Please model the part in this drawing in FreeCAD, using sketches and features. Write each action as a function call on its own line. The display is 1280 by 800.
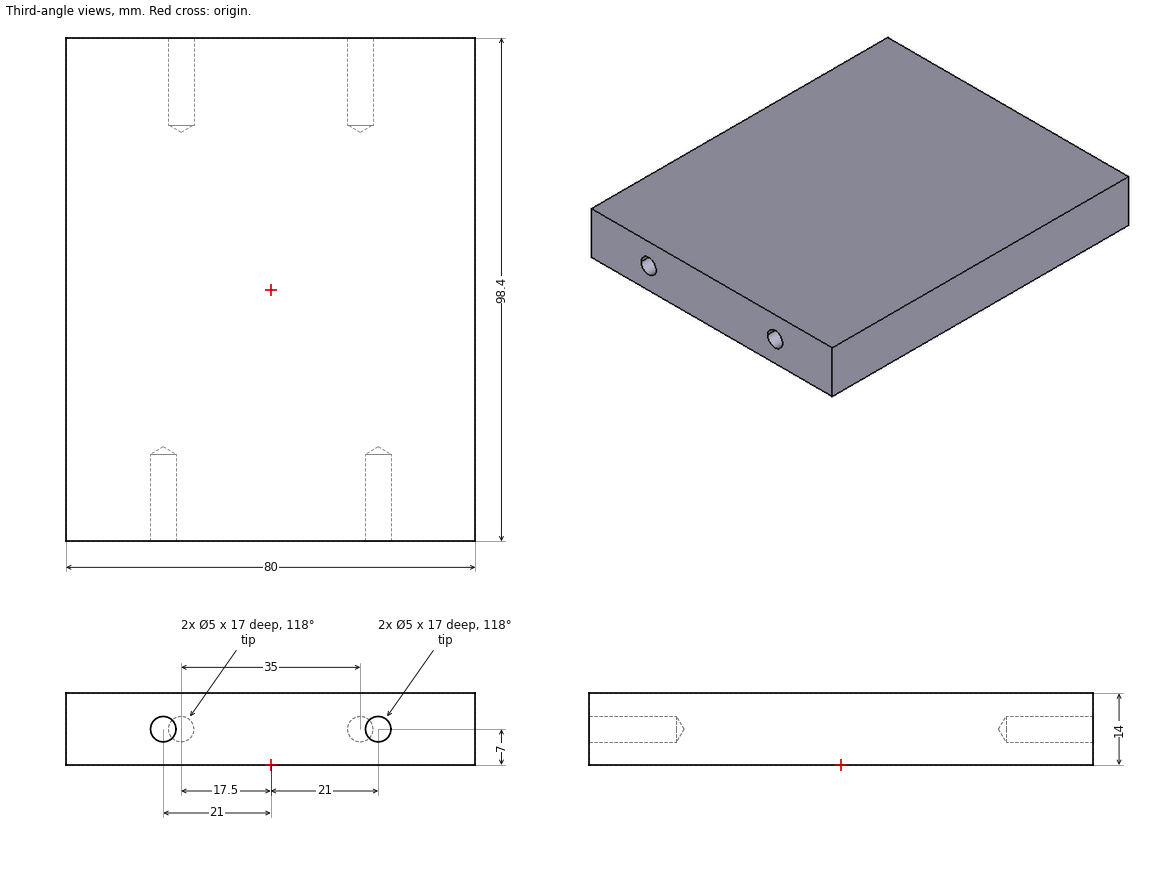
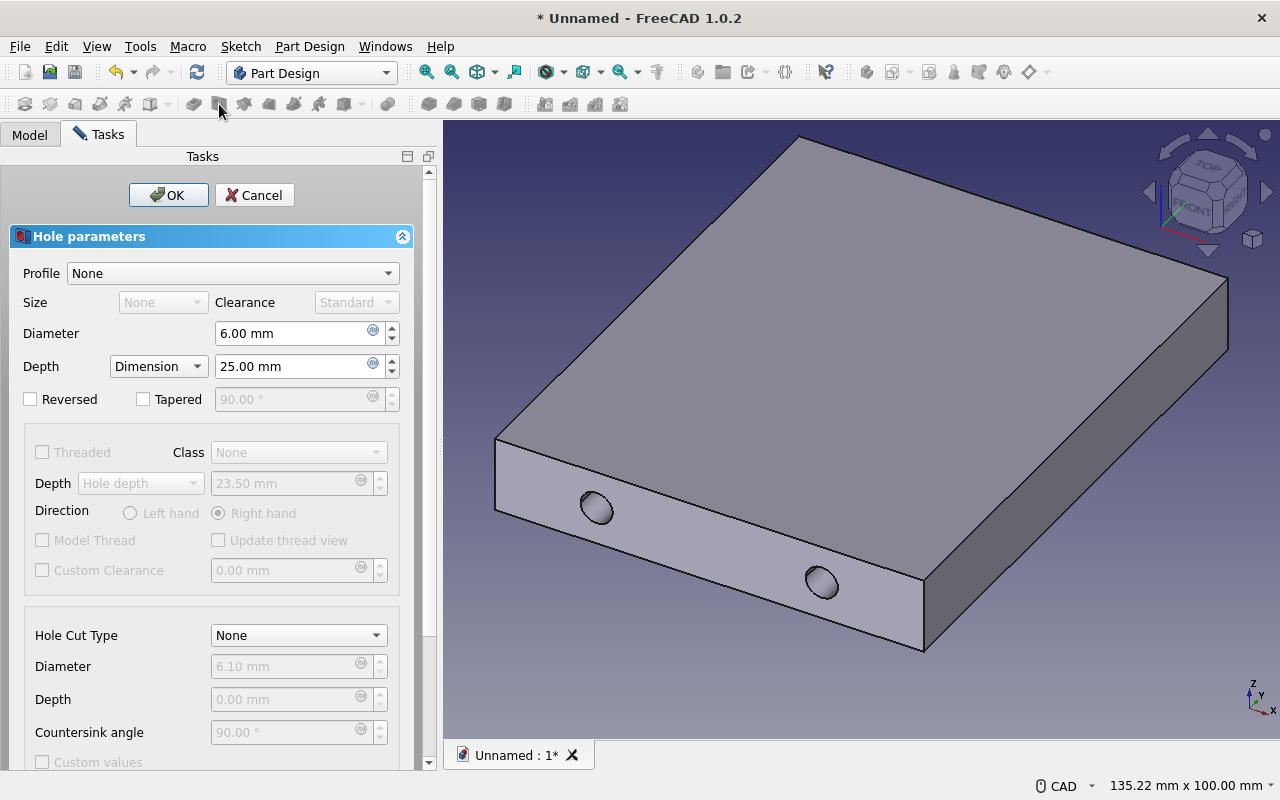
triple_click(300, 334)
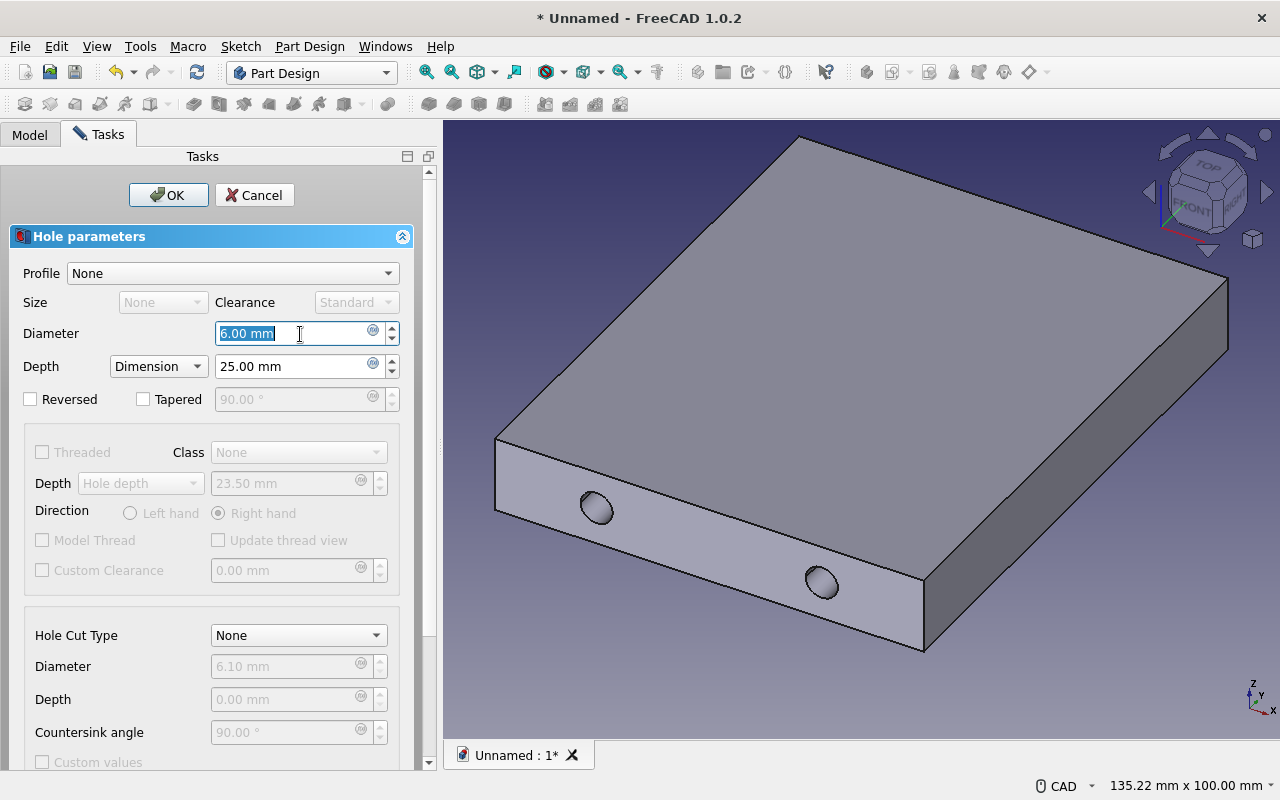
text(5)
key(Tab)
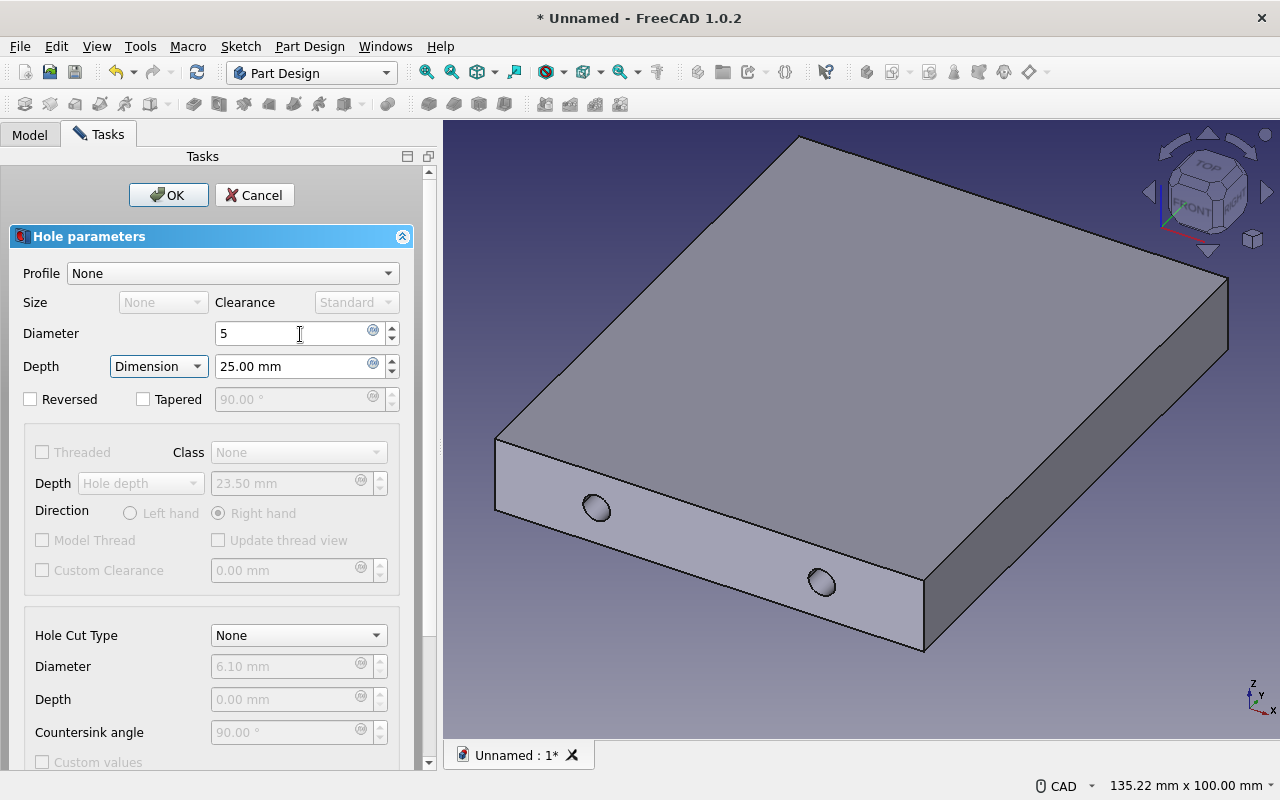
triple_click(300, 366)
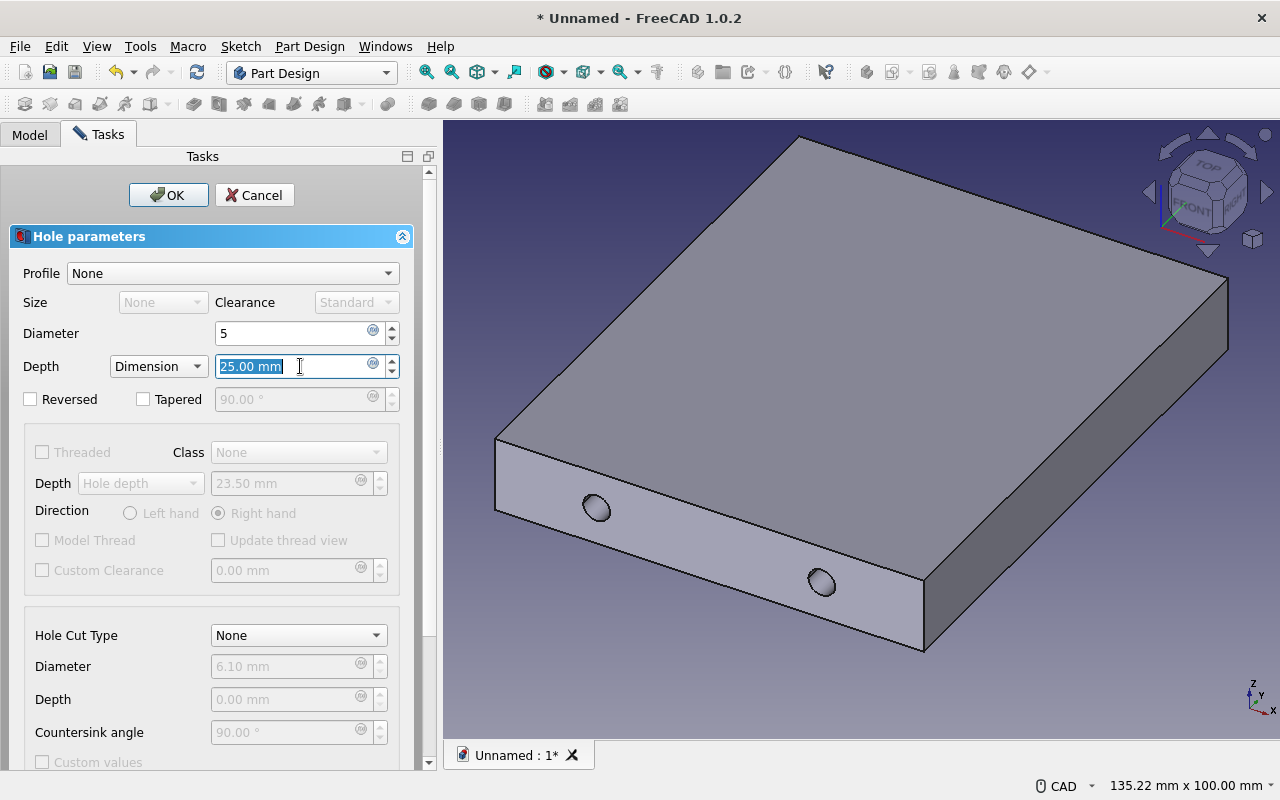
text(17)
key(Tab)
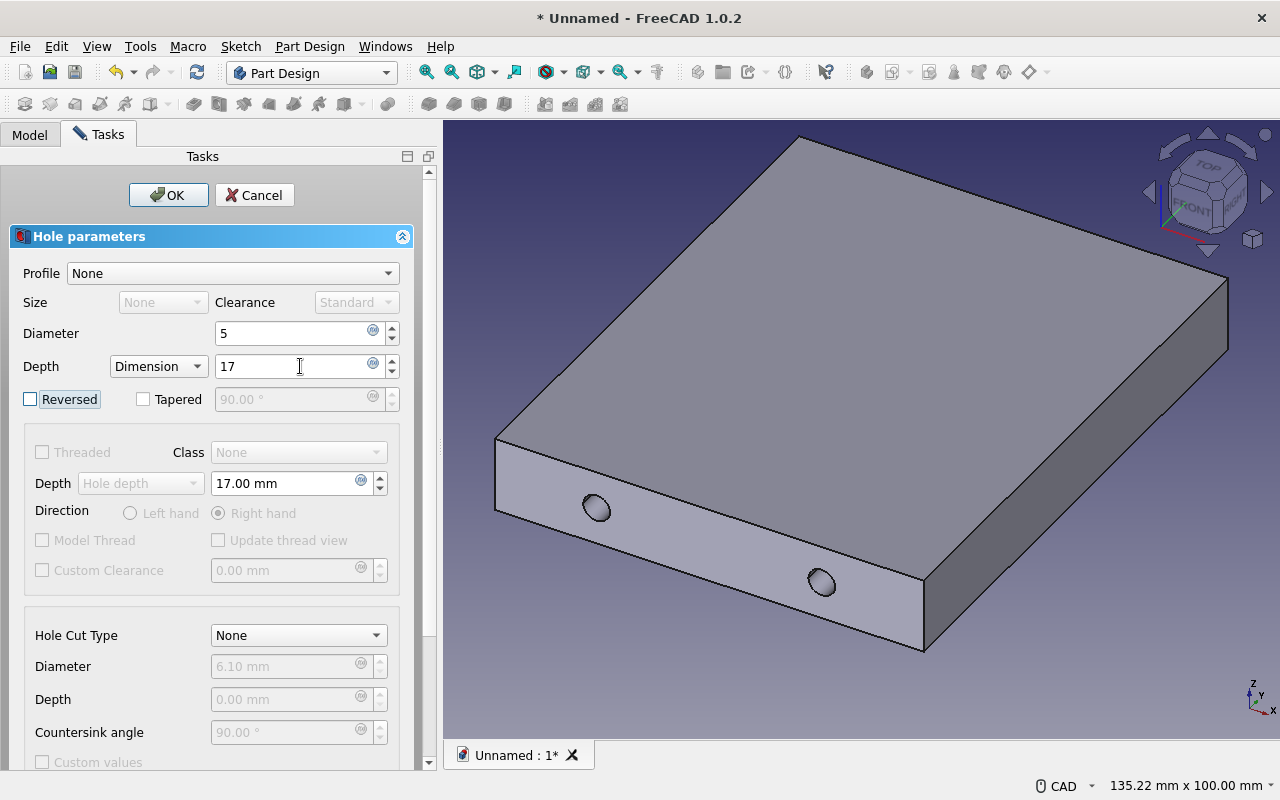
click(169, 195)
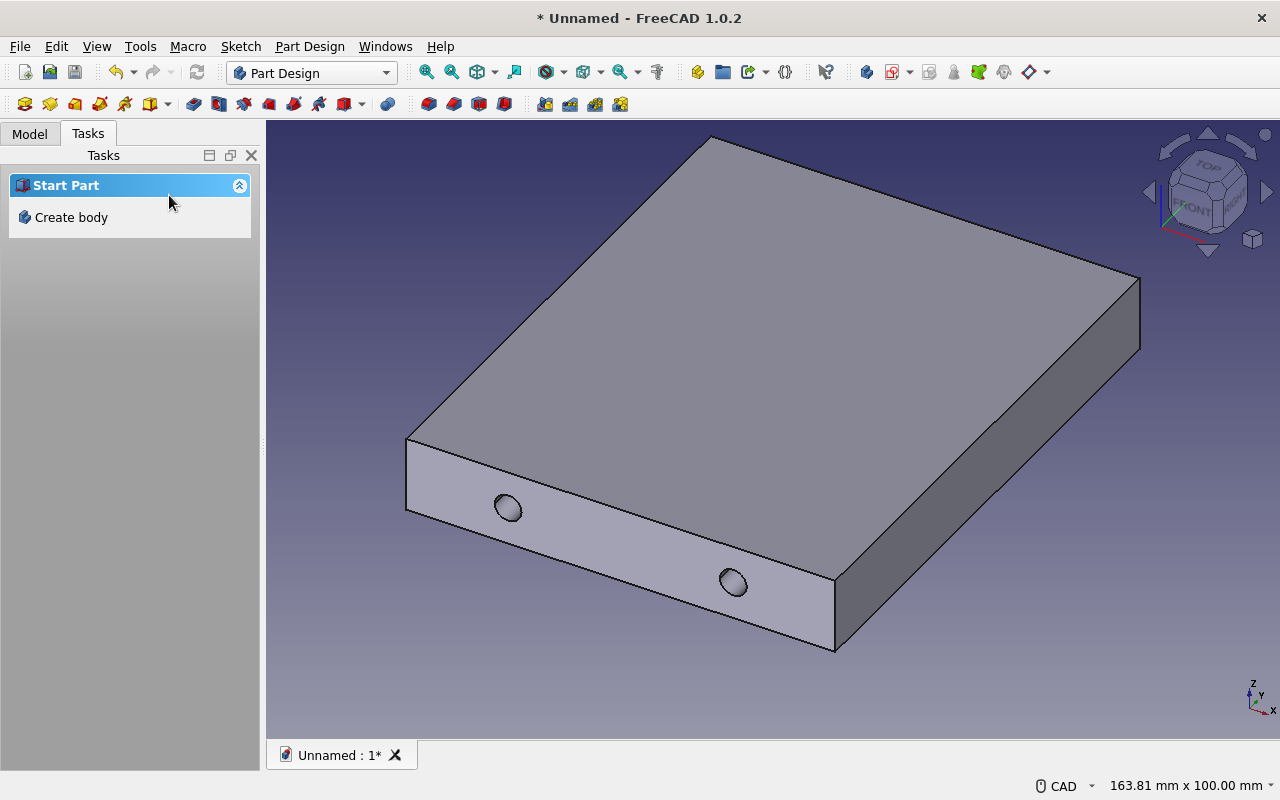
key(4)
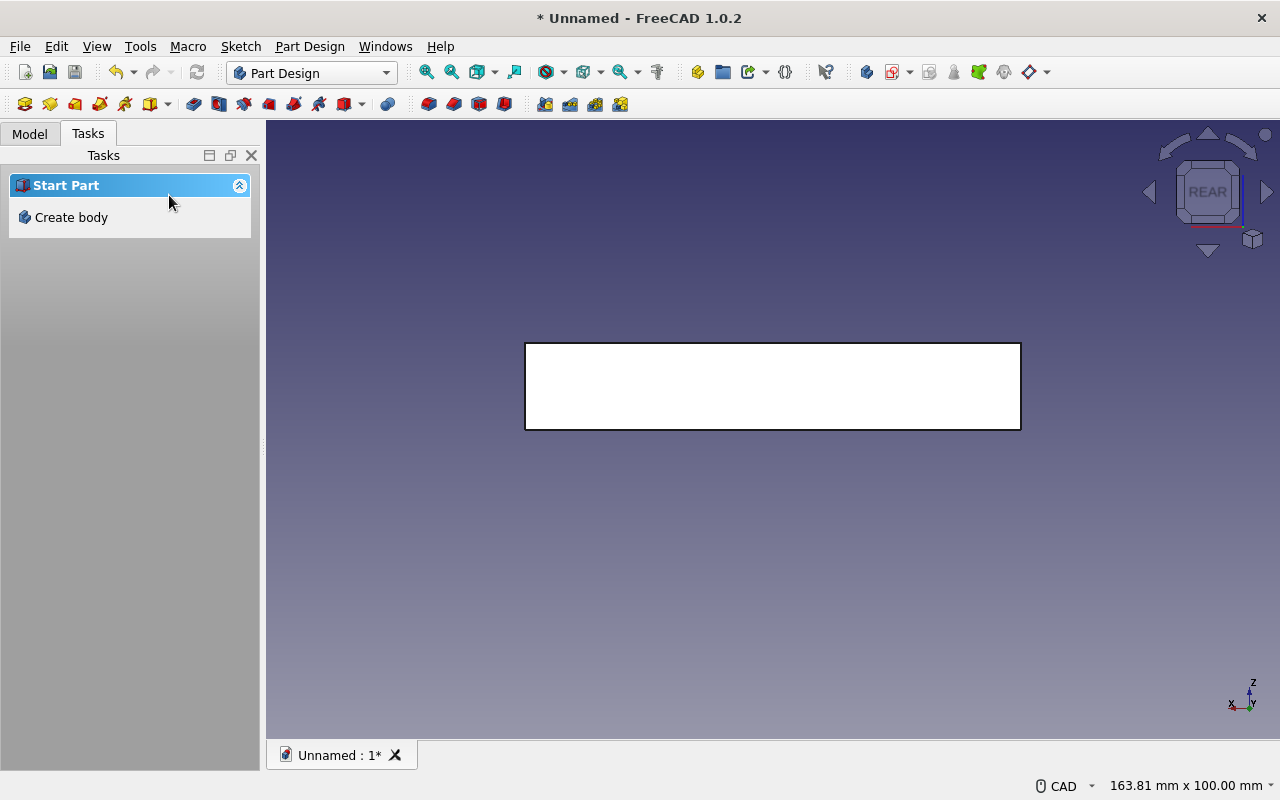
click(632, 385)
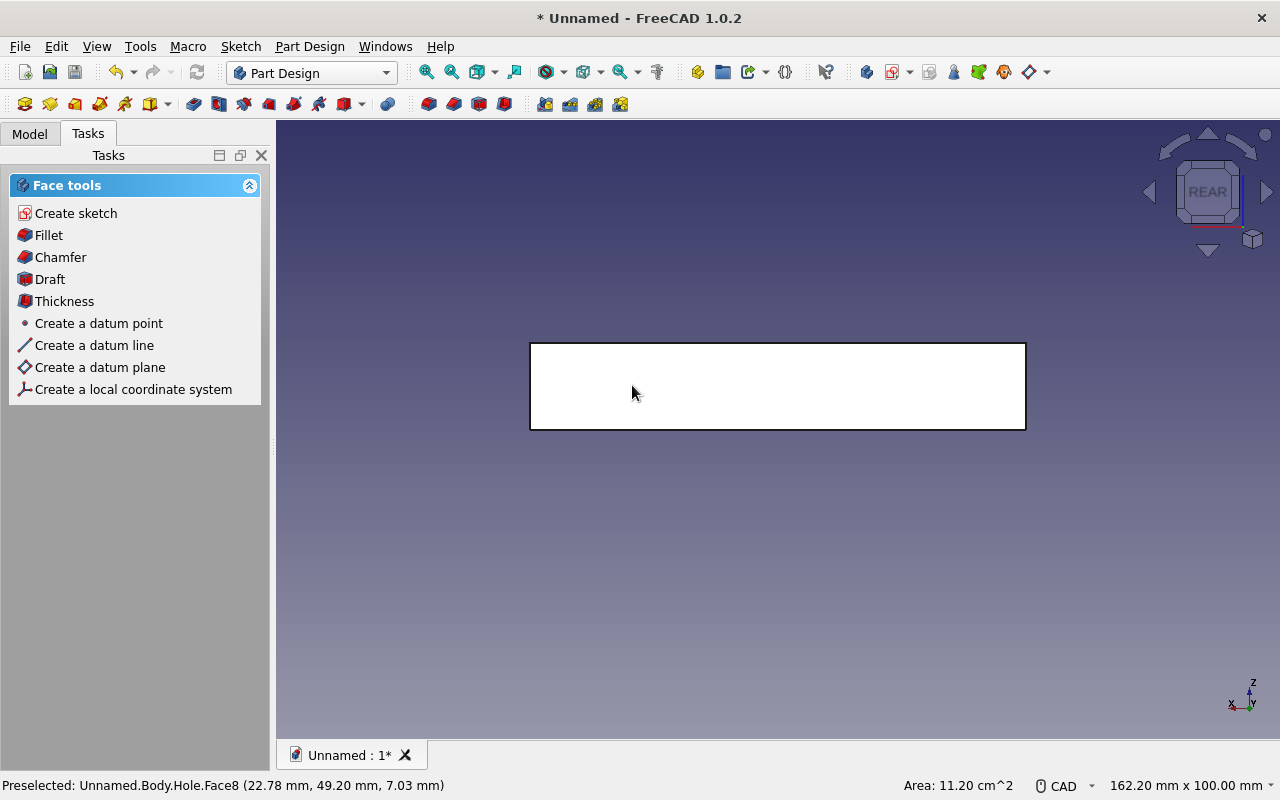
click(892, 72)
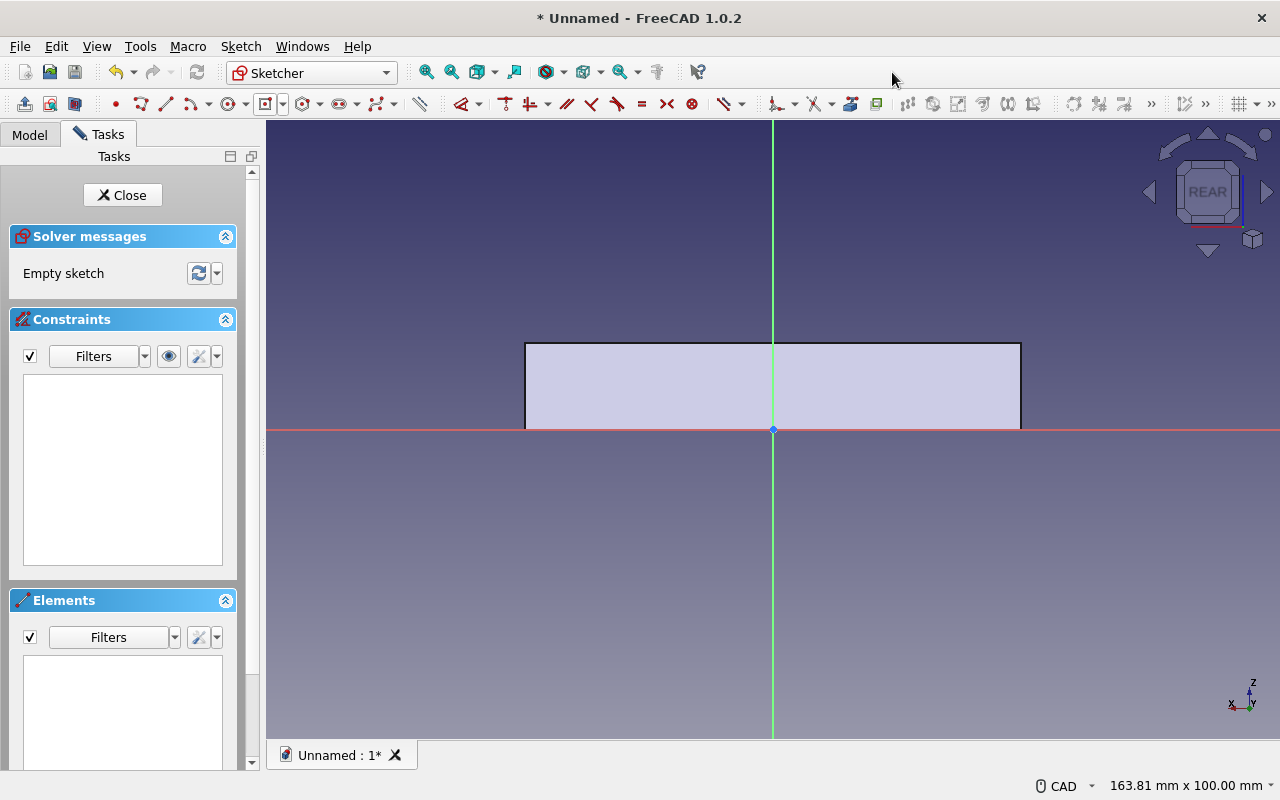
scroll(829, 376, up, 4)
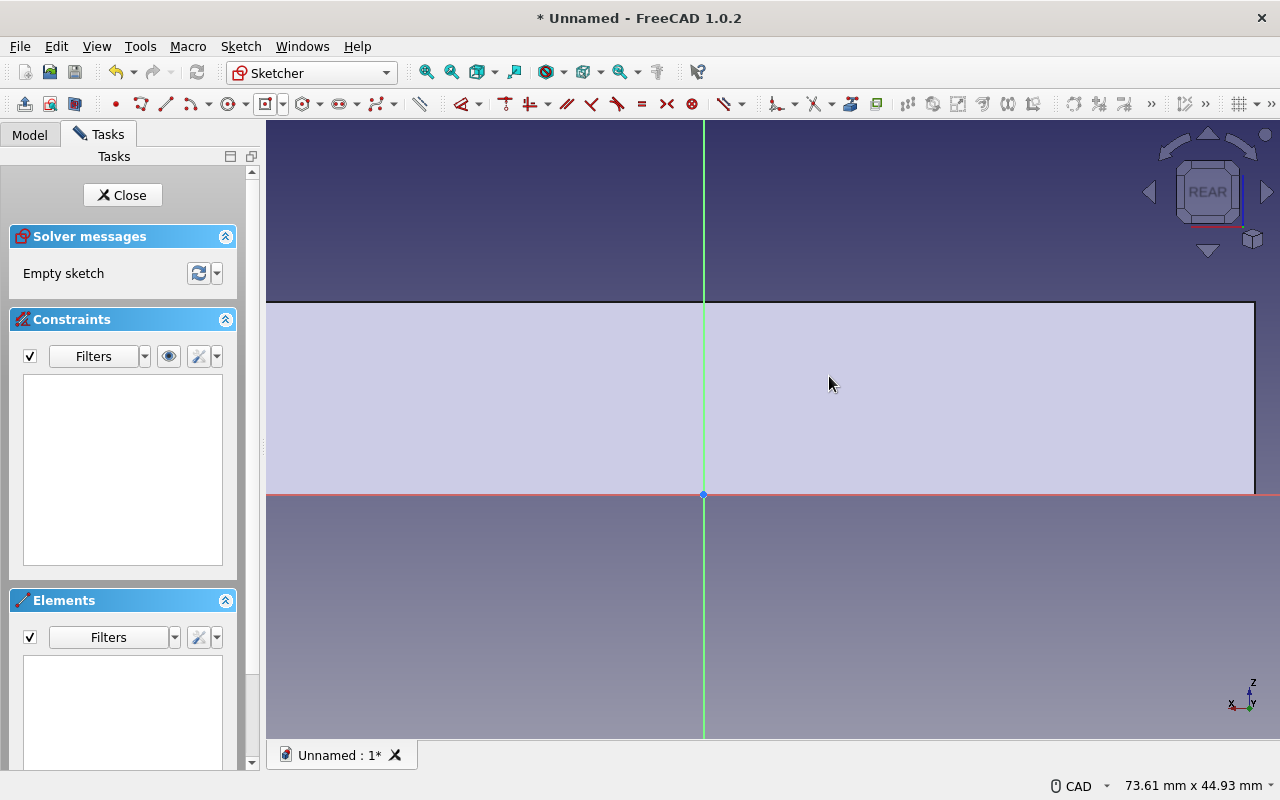
click(228, 104)